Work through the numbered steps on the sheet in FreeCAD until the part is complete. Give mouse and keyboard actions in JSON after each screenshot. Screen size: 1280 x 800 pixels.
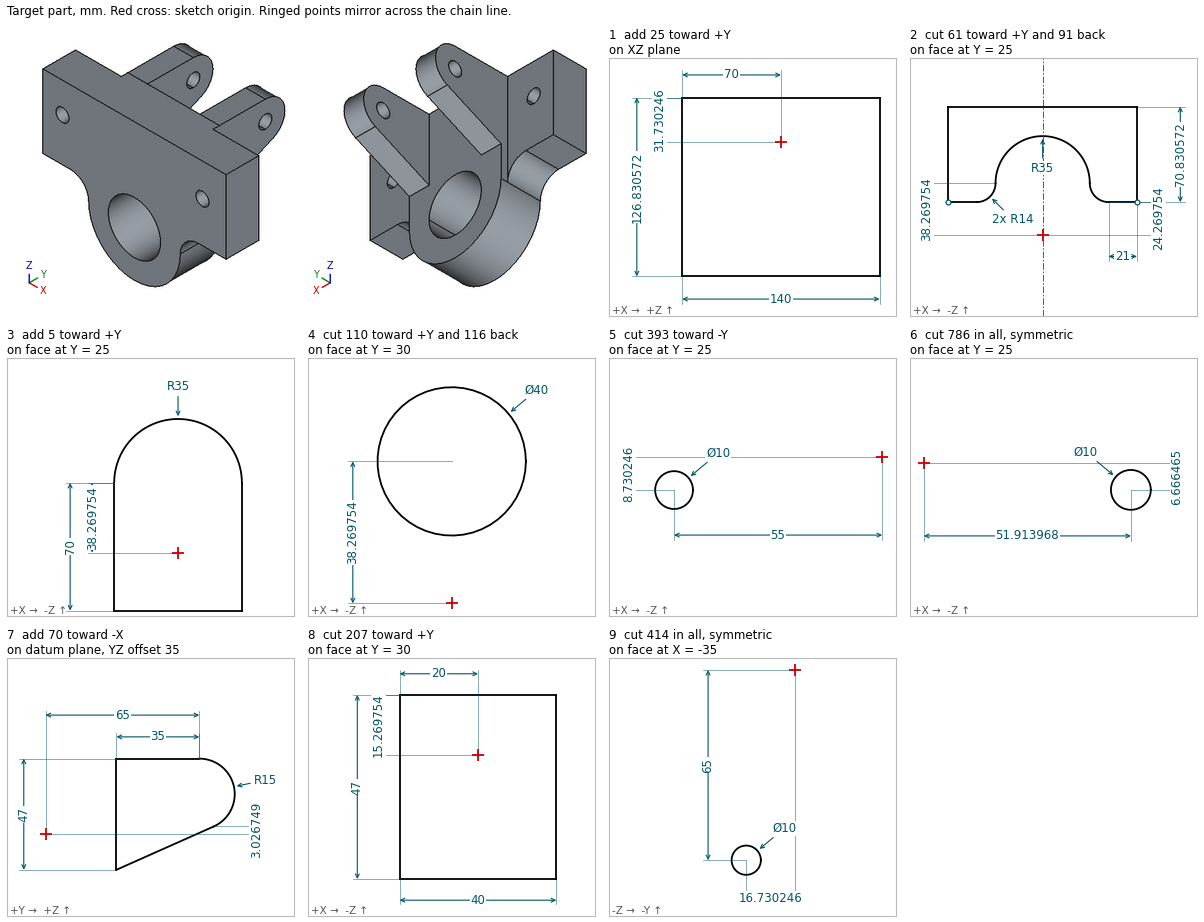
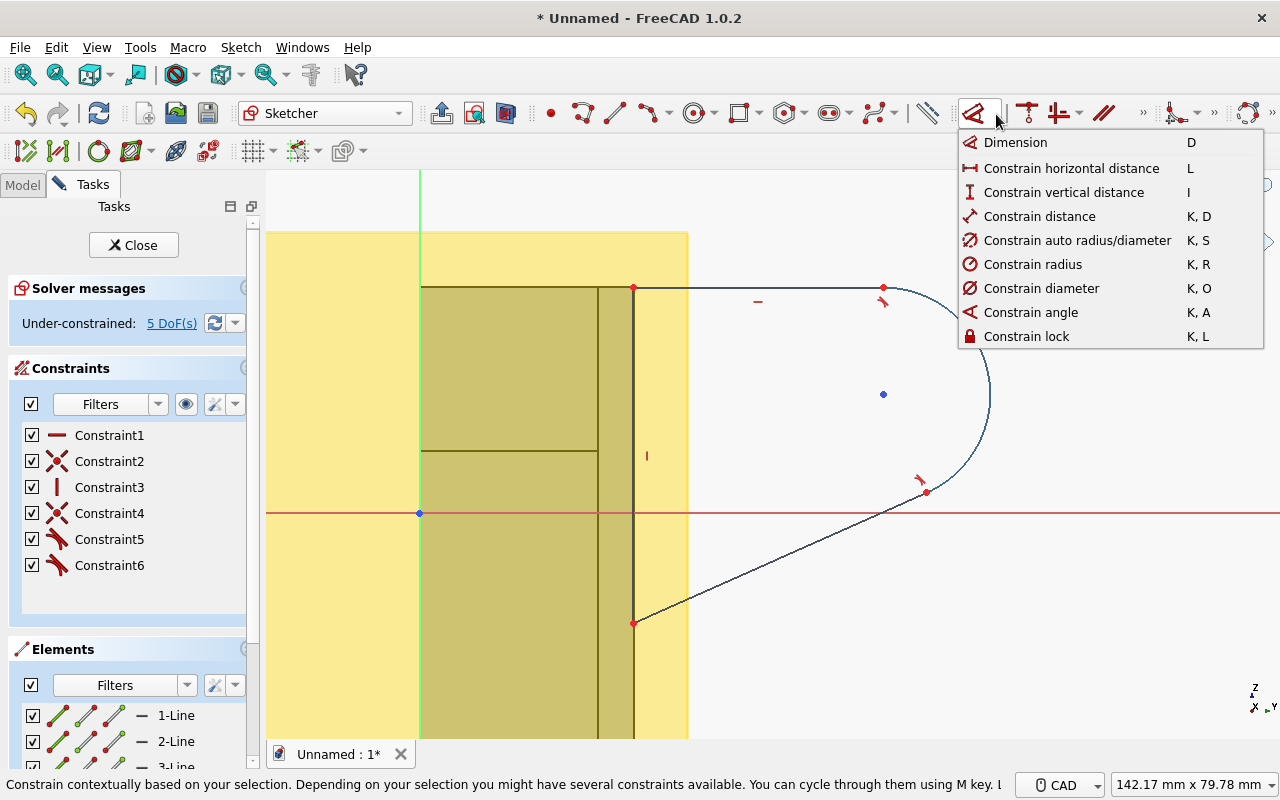
{"action": "left_click", "coordinate": [1111, 264]}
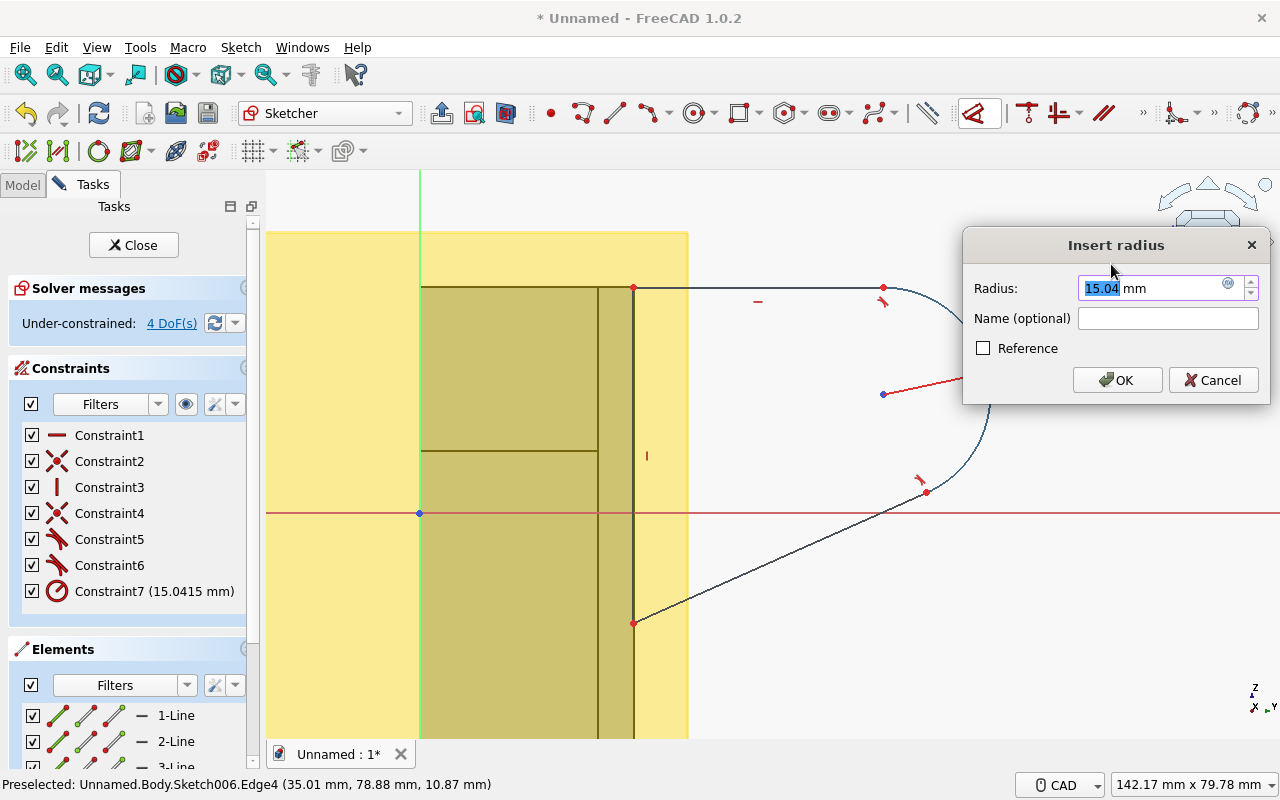
{"action": "type", "text": "15"}
{"action": "key", "text": "Return"}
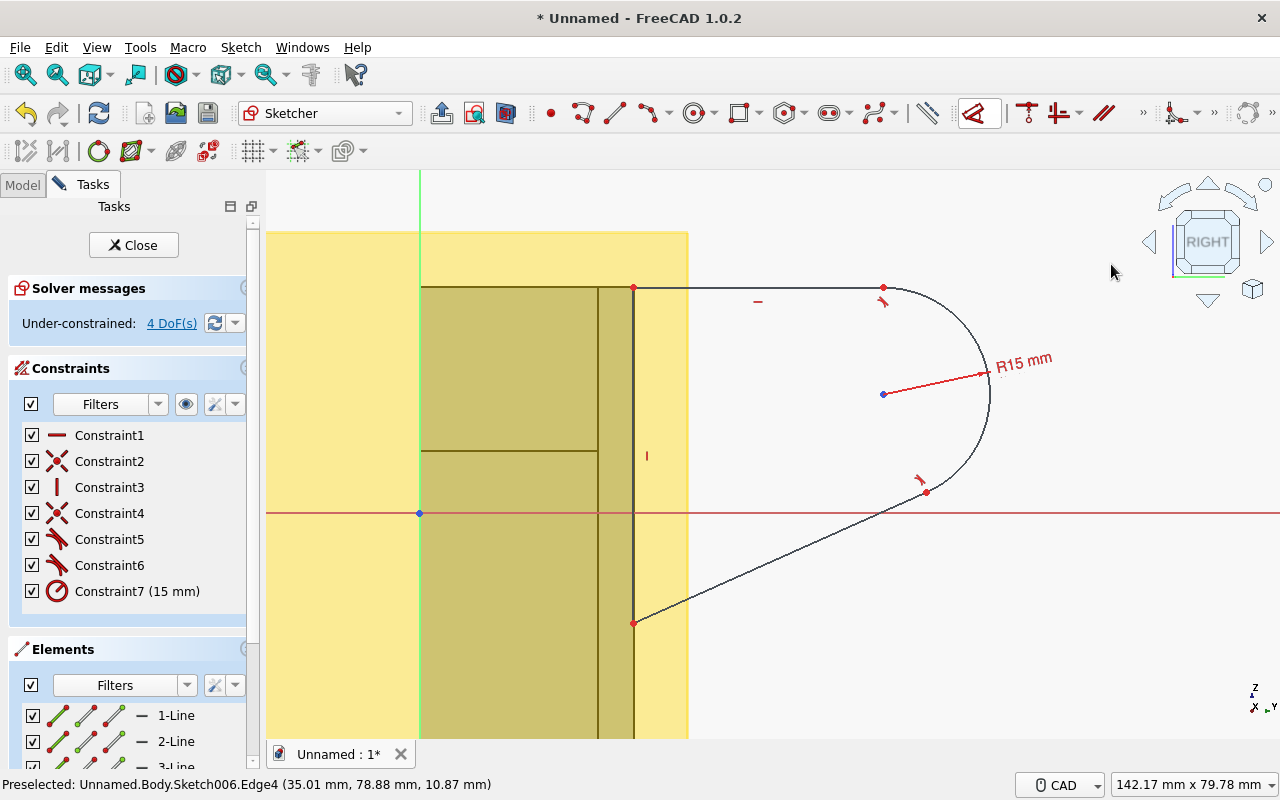
{"action": "left_click", "coordinate": [808, 288]}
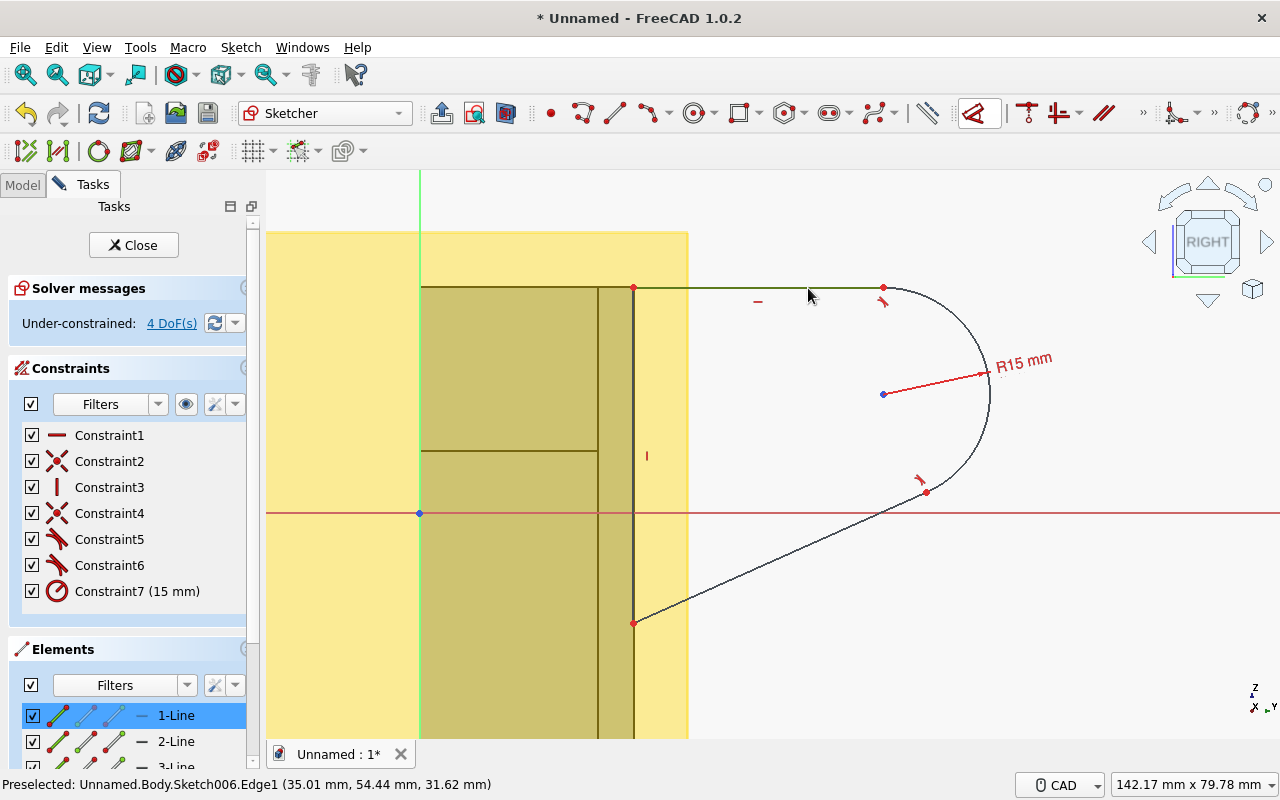
{"action": "left_click", "coordinate": [996, 114]}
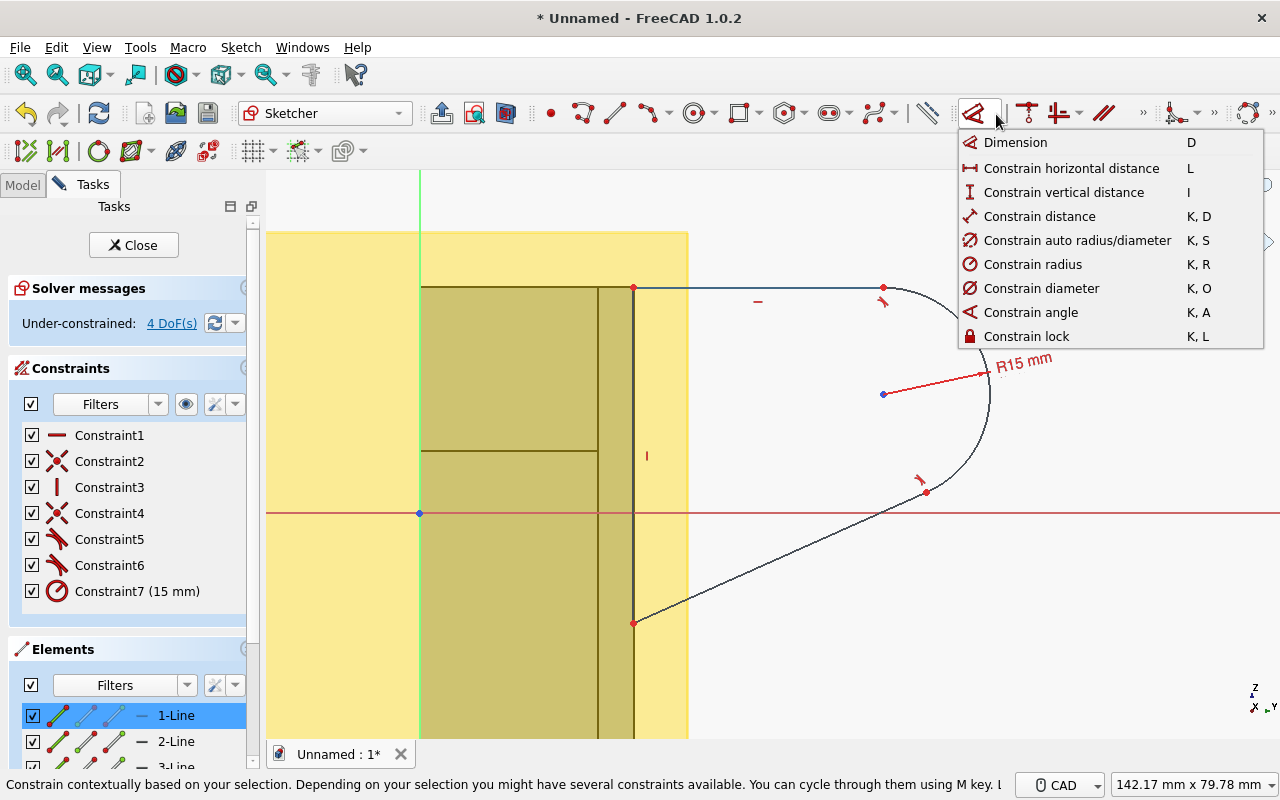
{"action": "left_click", "coordinate": [1111, 168]}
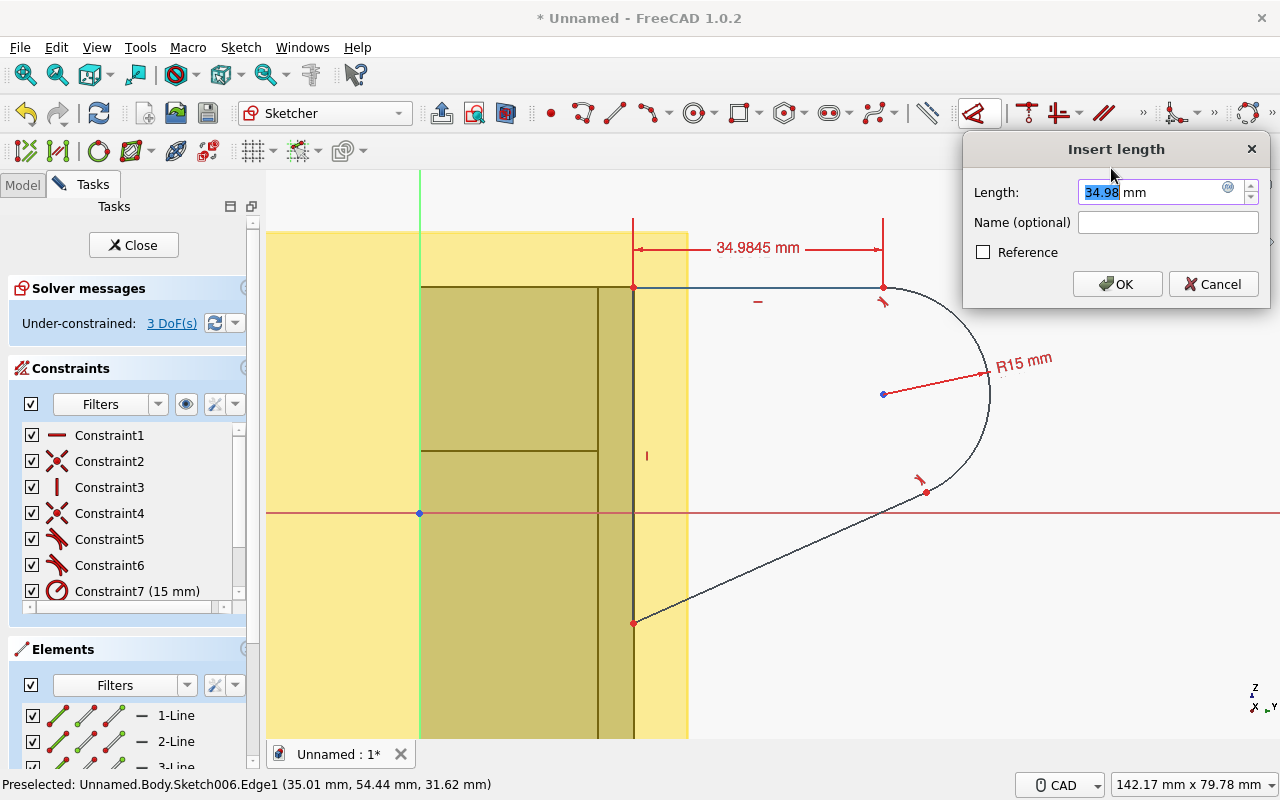
{"action": "type", "text": "35"}
{"action": "key", "text": "Return"}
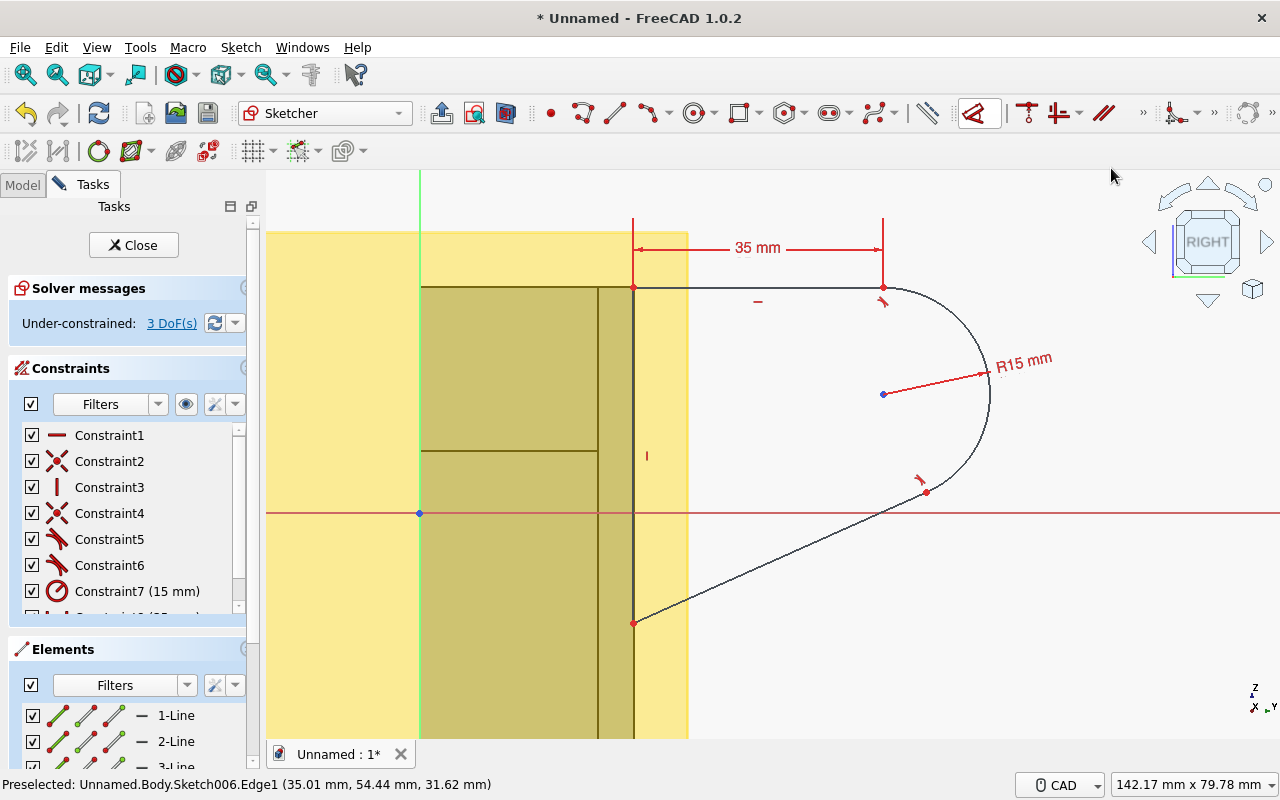
{"action": "left_click", "coordinate": [633, 388]}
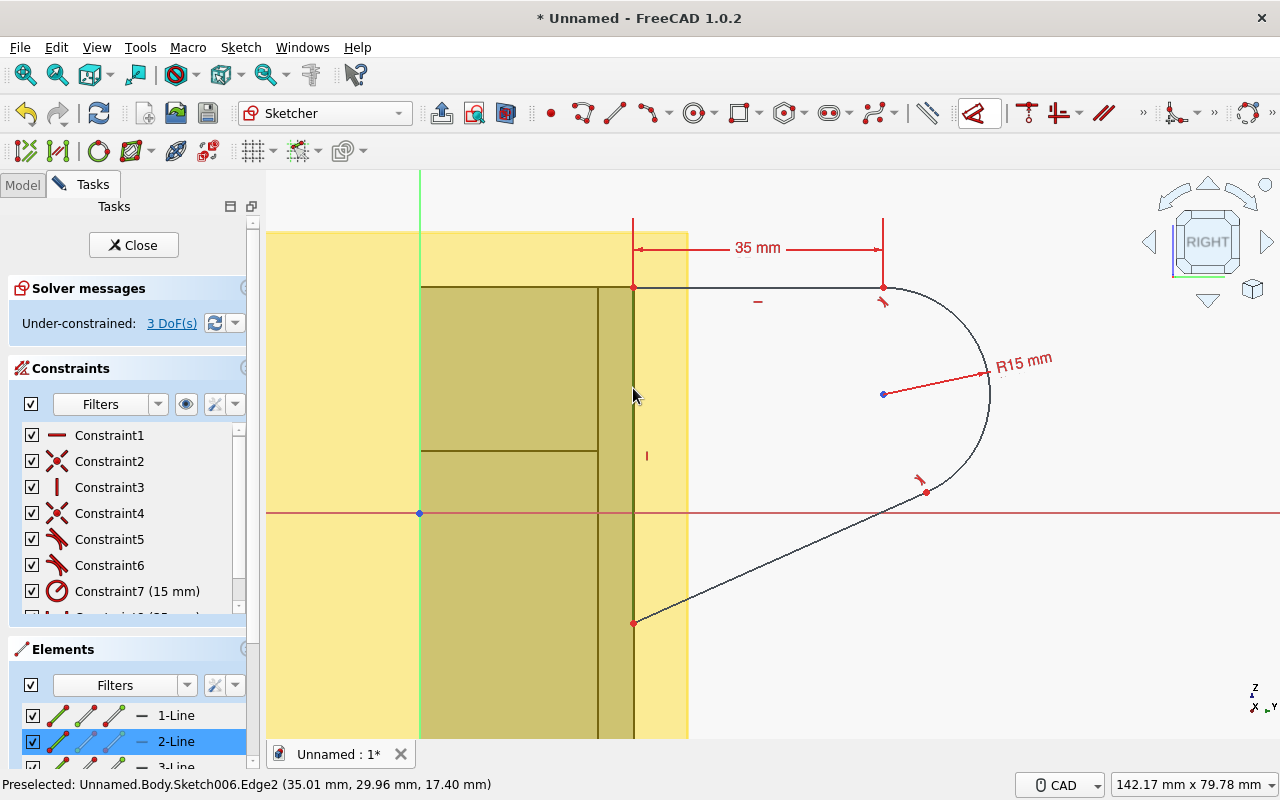
{"action": "left_click", "coordinate": [996, 114]}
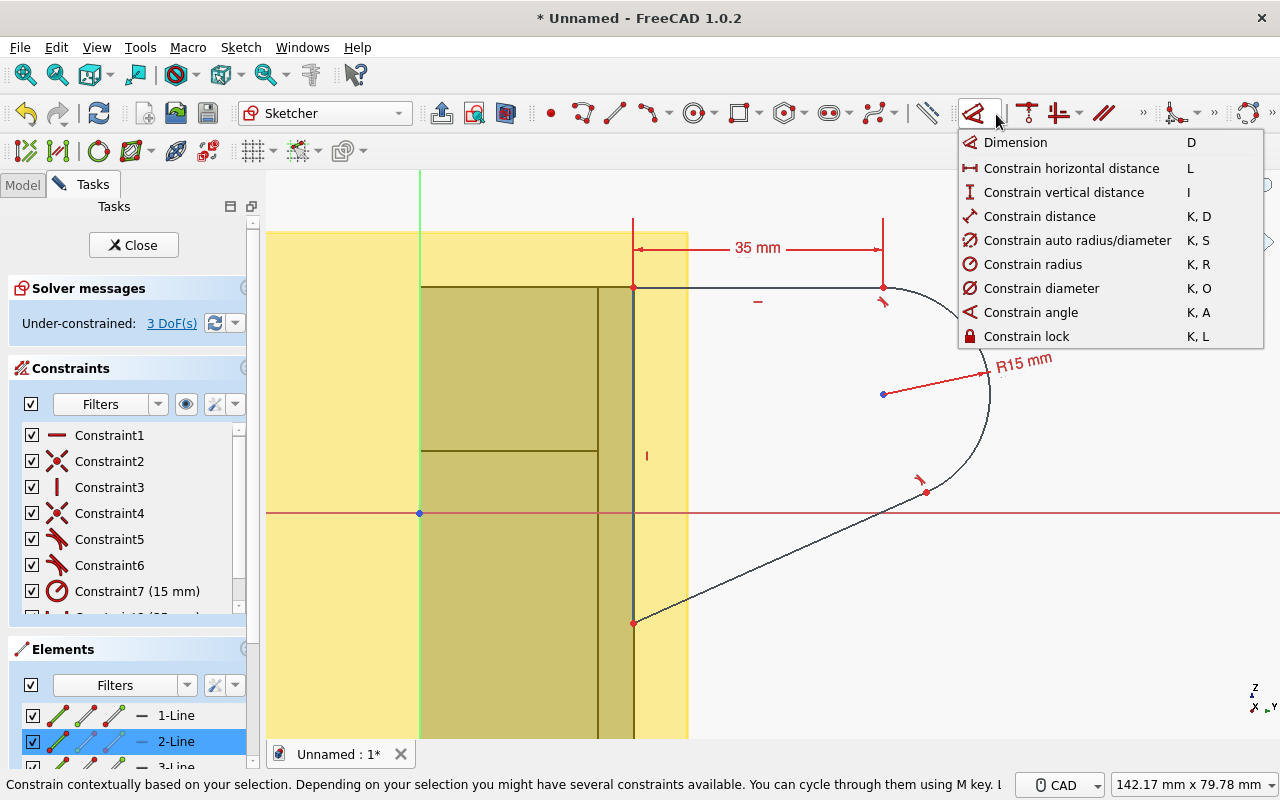
{"action": "left_click", "coordinate": [1111, 192]}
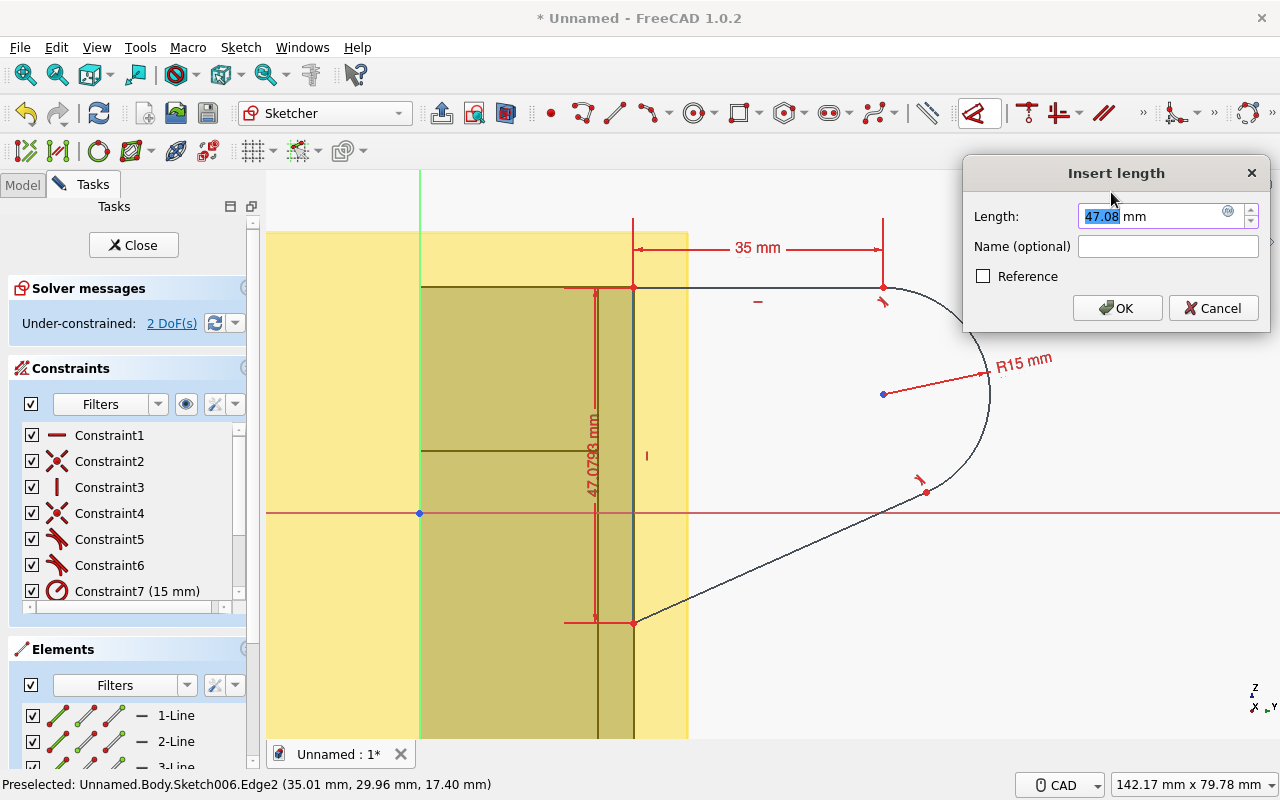
{"action": "type", "text": "47"}
{"action": "key", "text": "Return"}